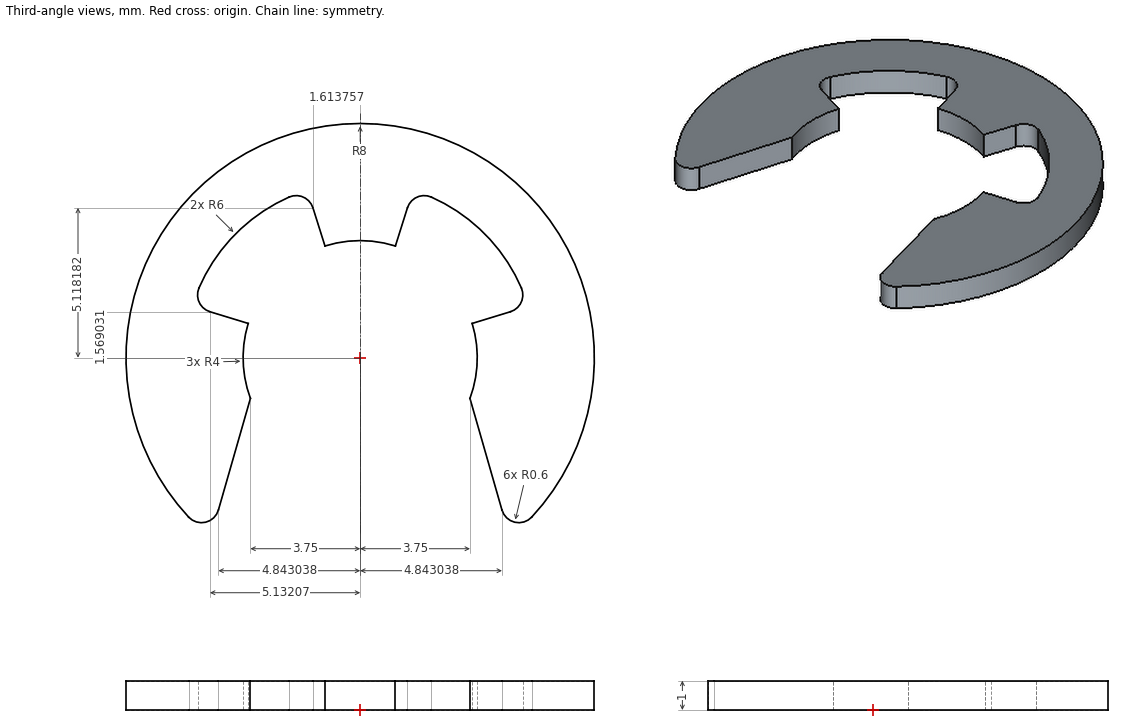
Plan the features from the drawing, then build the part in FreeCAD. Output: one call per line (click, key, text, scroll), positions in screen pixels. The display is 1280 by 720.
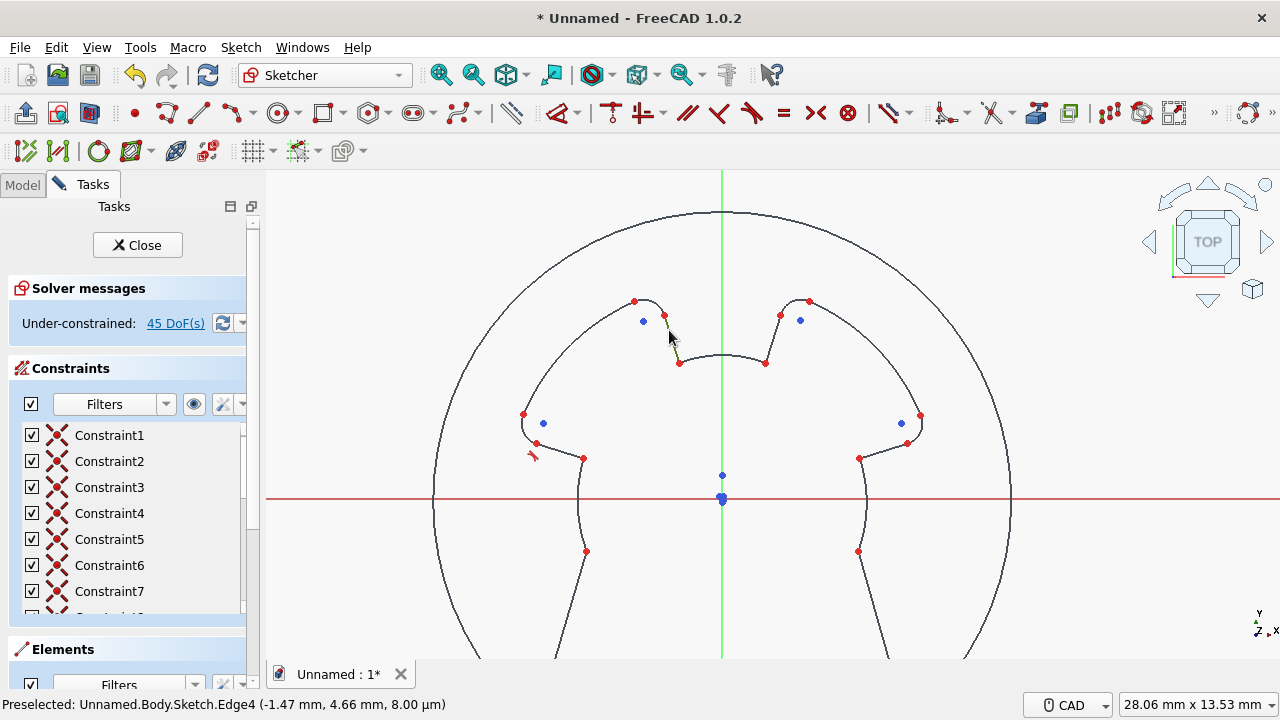
scroll(659, 306, up, 2)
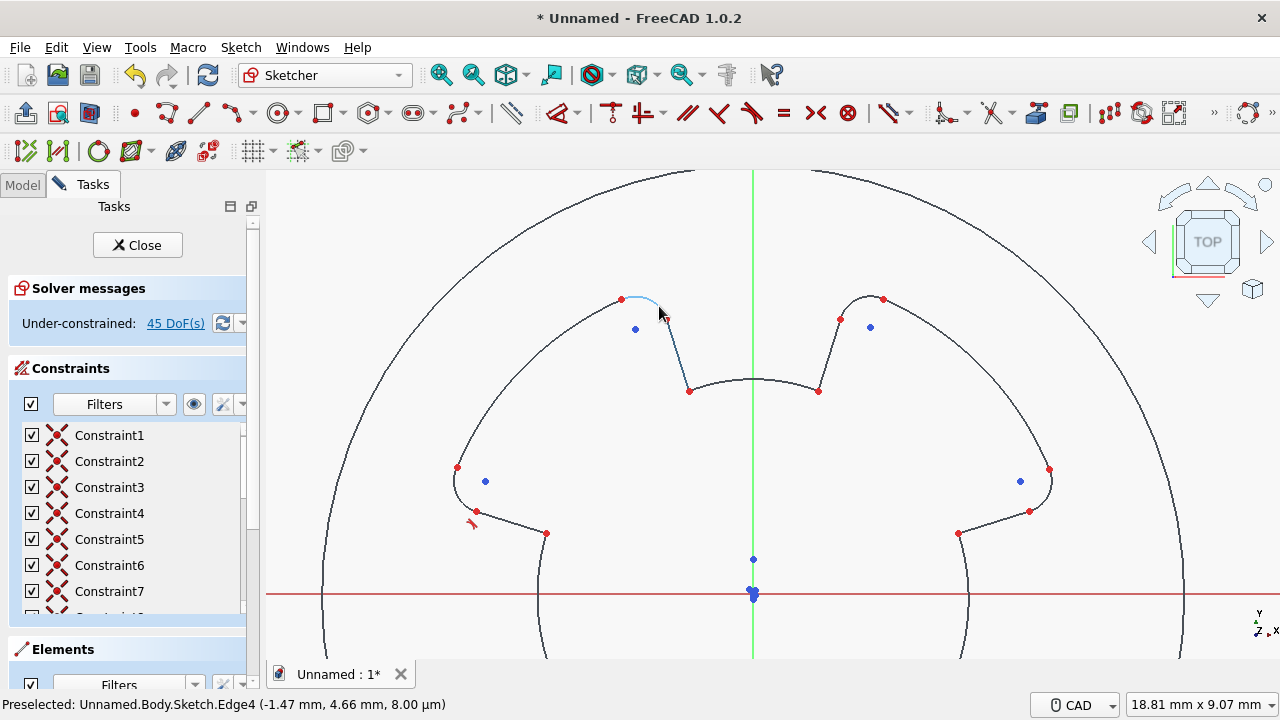
click(658, 306)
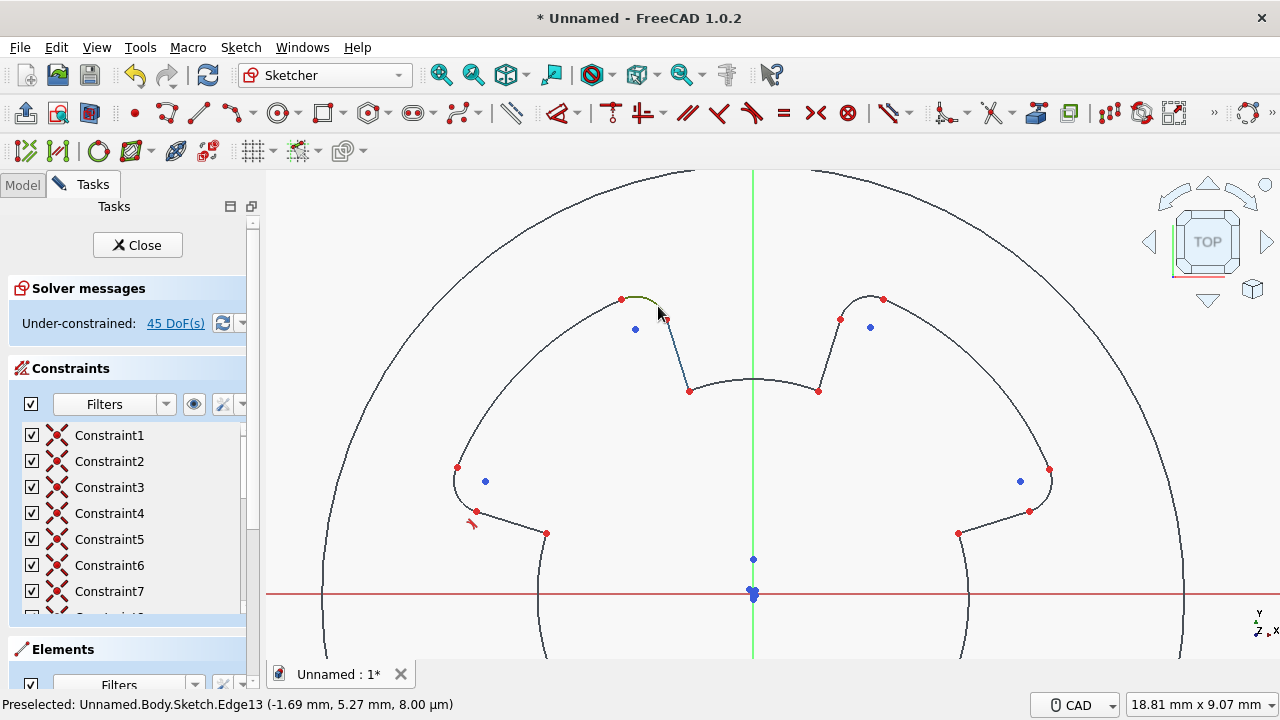
click(752, 114)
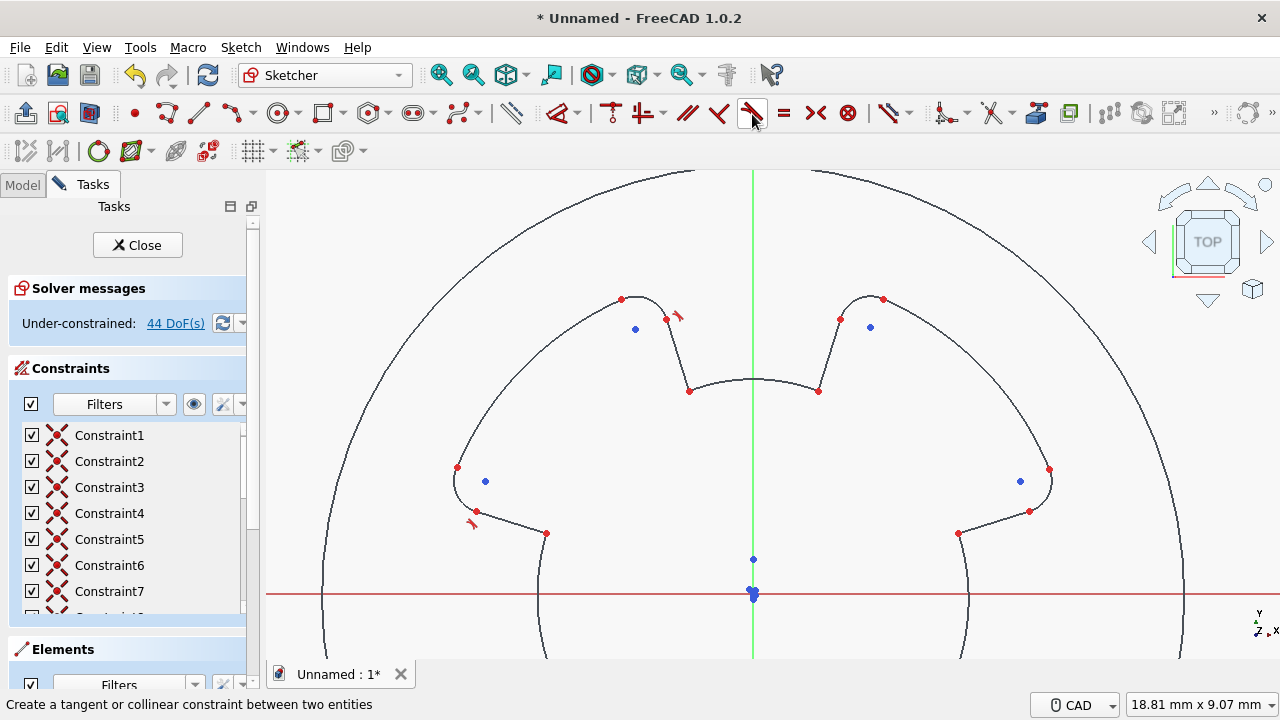
click(825, 370)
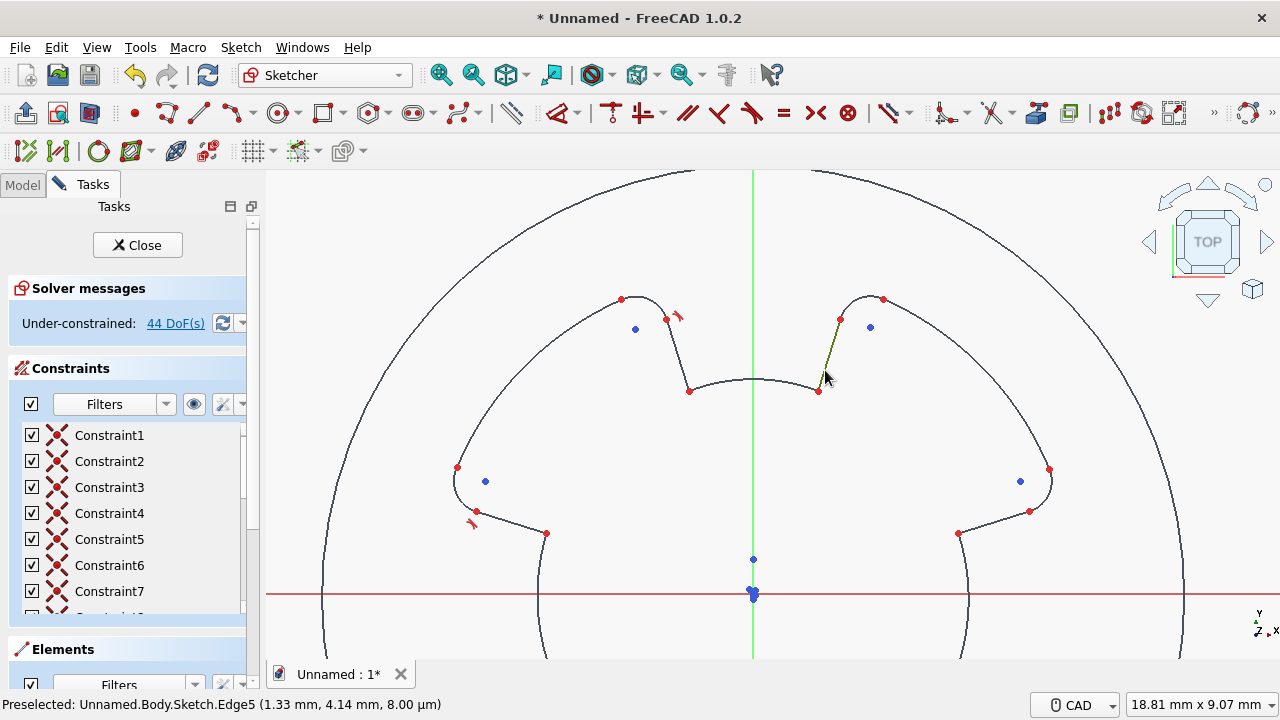
click(868, 296)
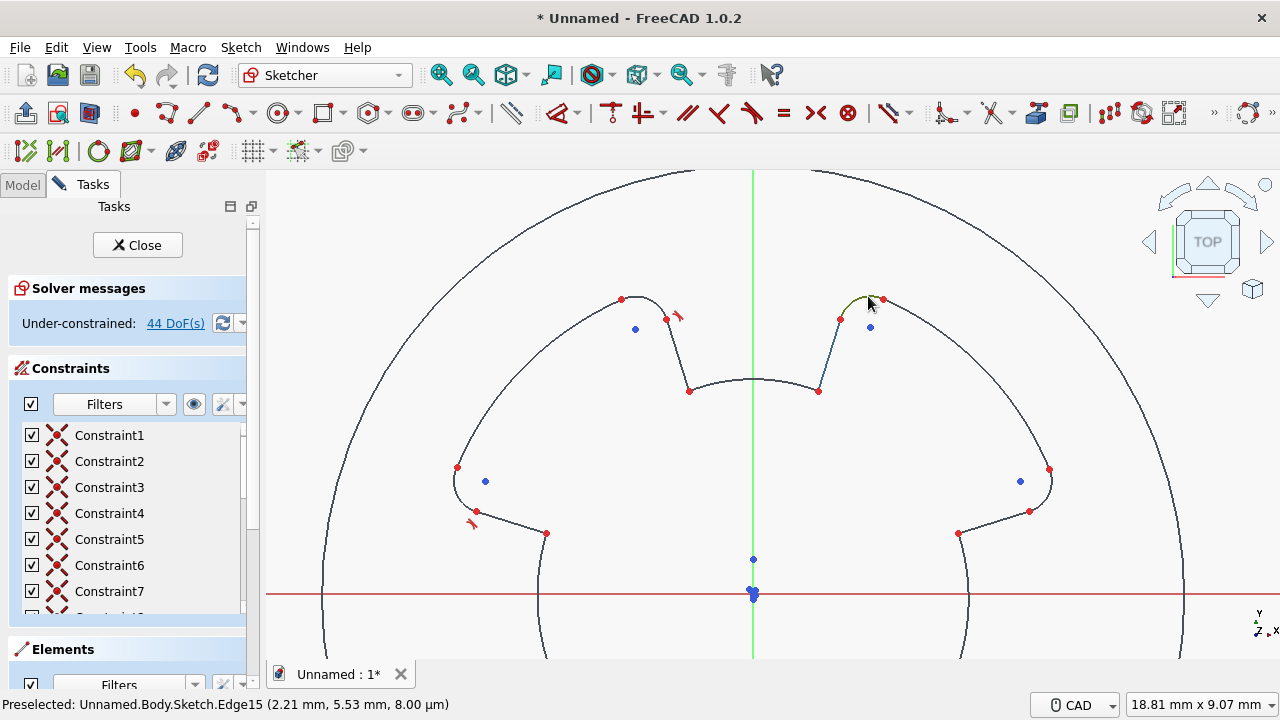
click(752, 114)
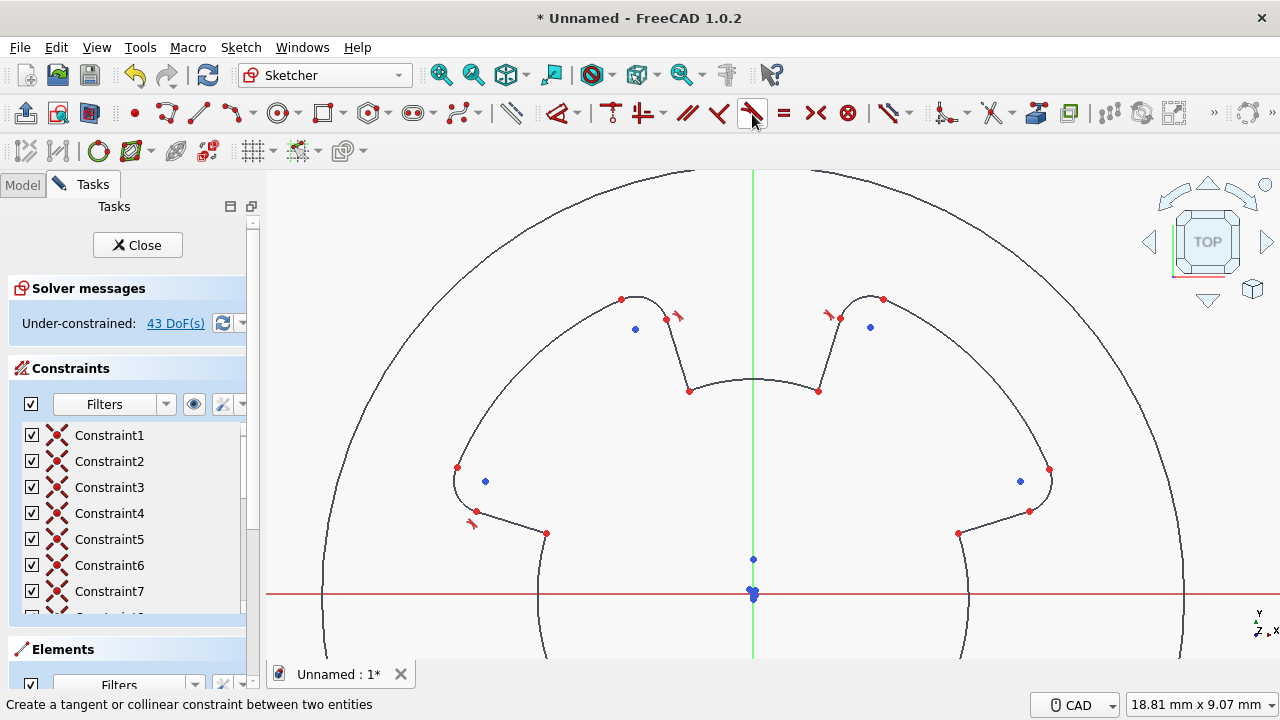
click(1008, 518)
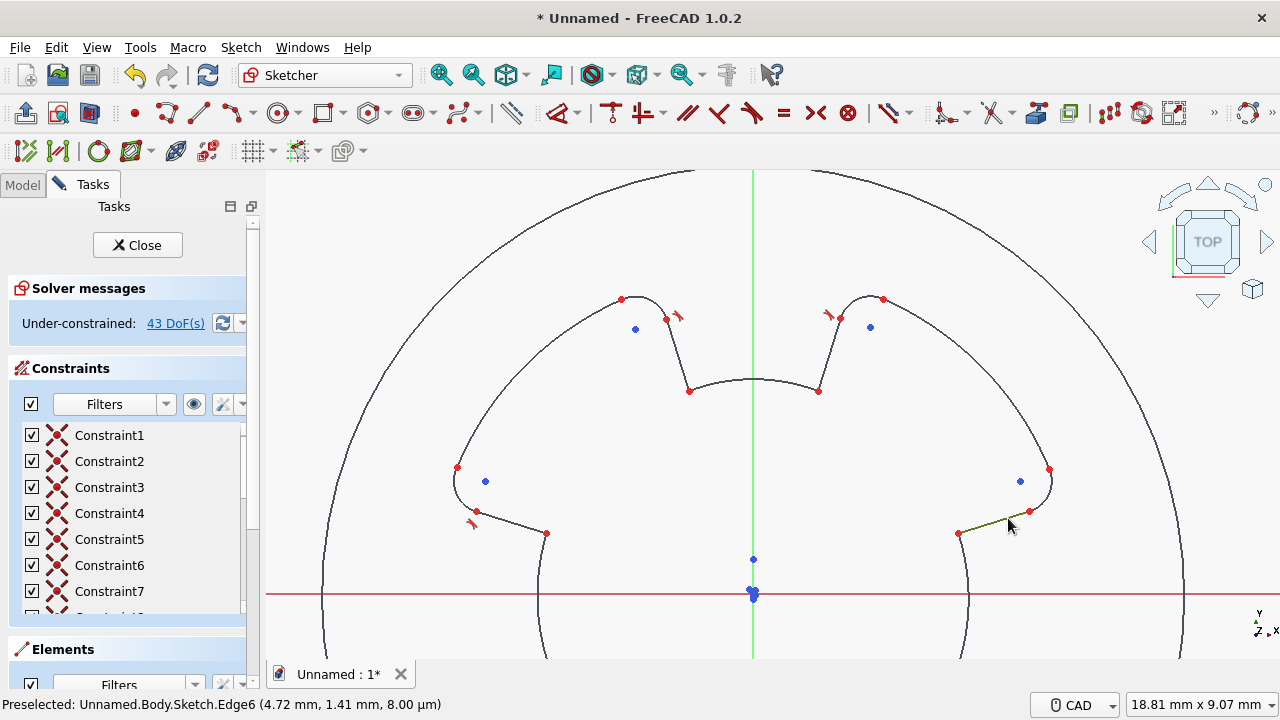
click(1043, 503)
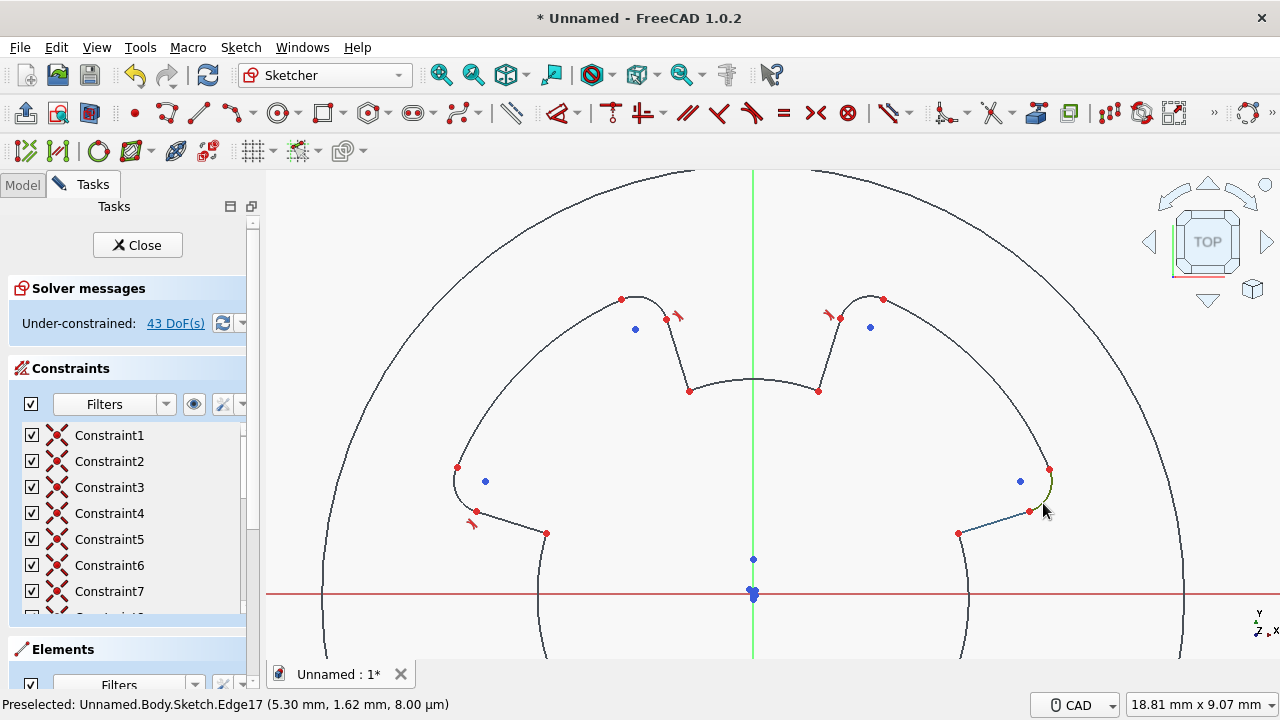
key(t)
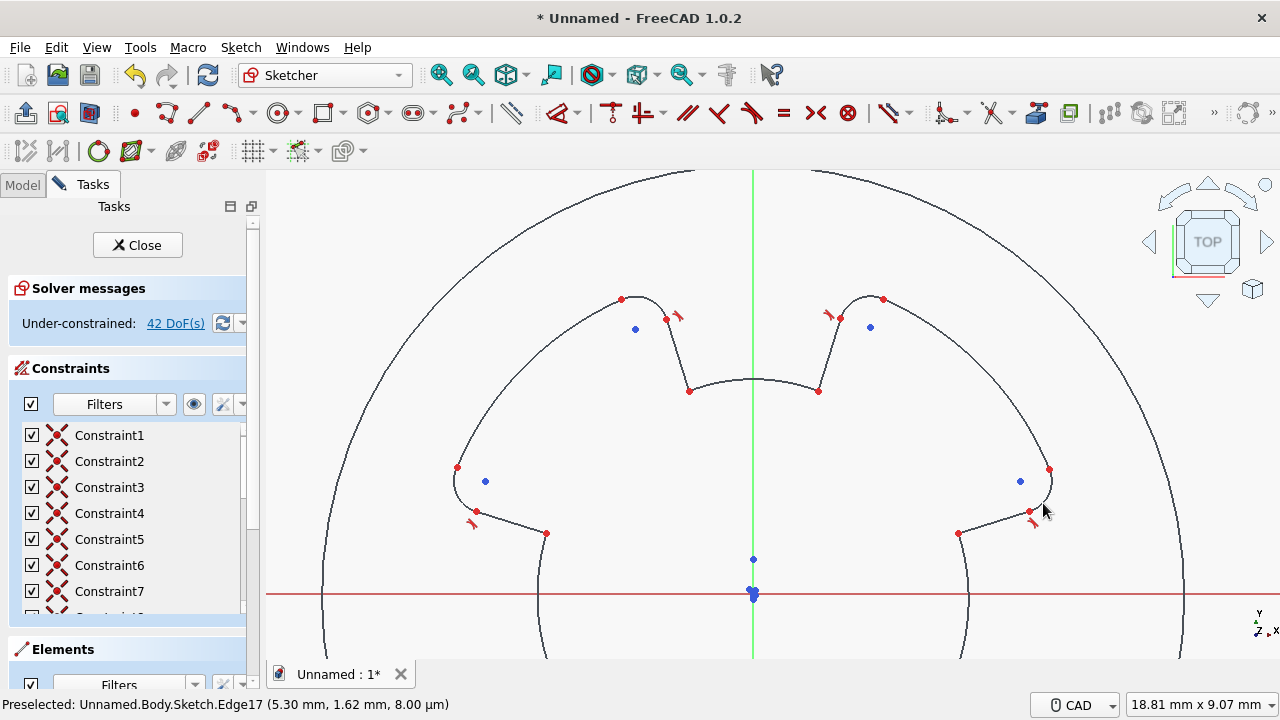
scroll(665, 320, down, 4)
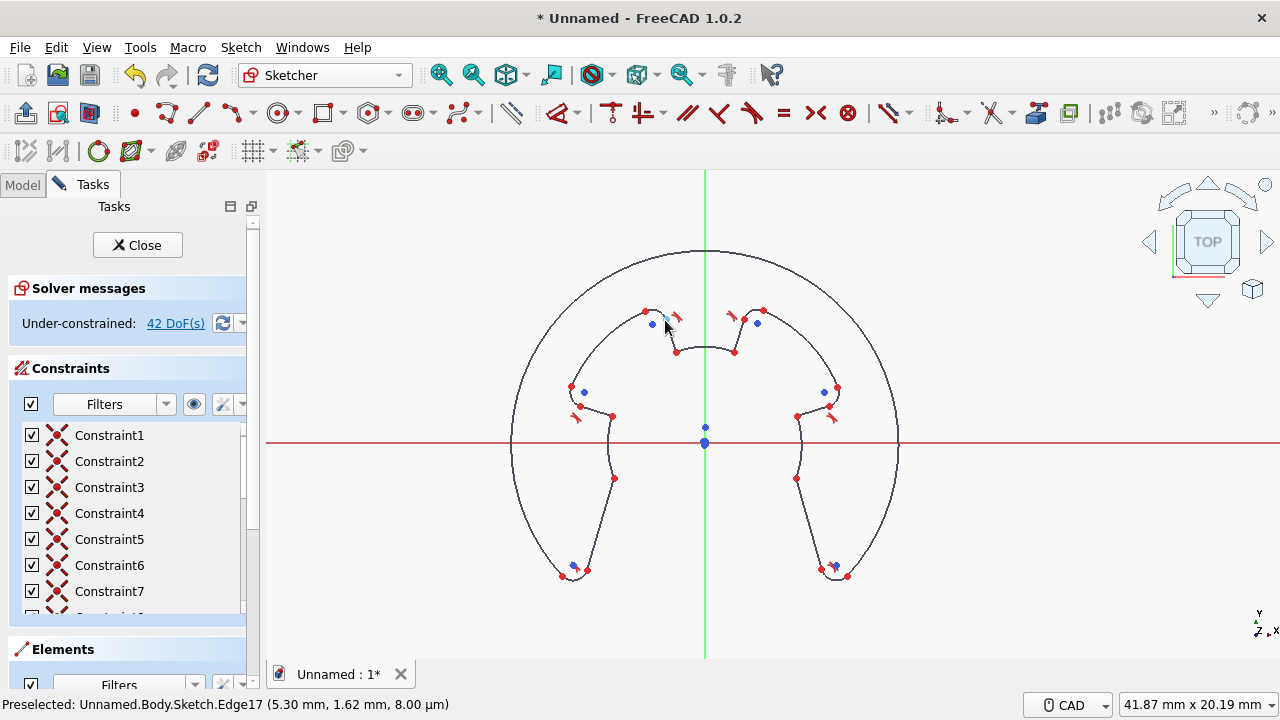
scroll(827, 577, up, 2)